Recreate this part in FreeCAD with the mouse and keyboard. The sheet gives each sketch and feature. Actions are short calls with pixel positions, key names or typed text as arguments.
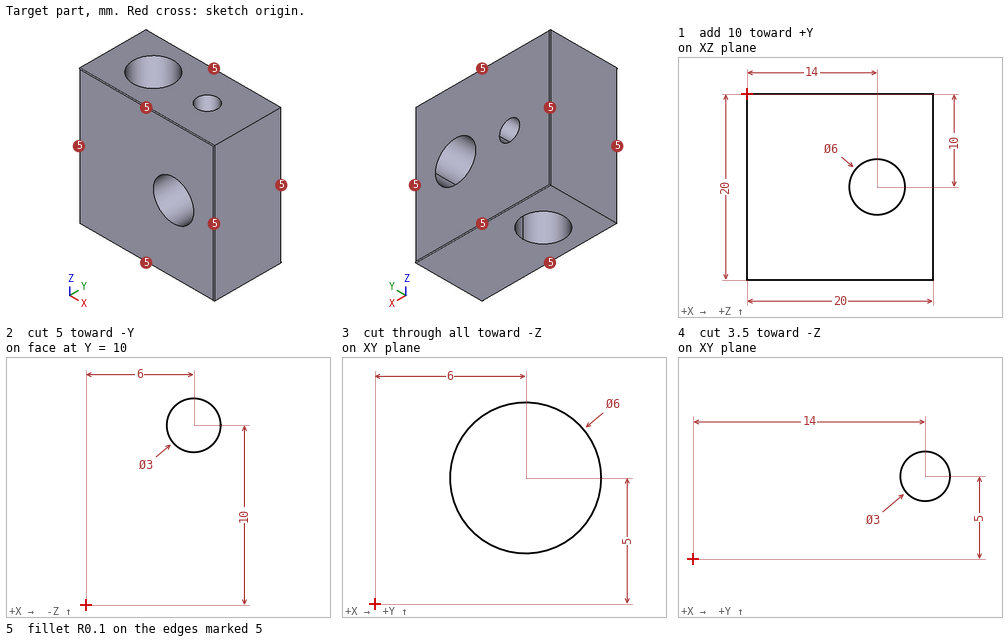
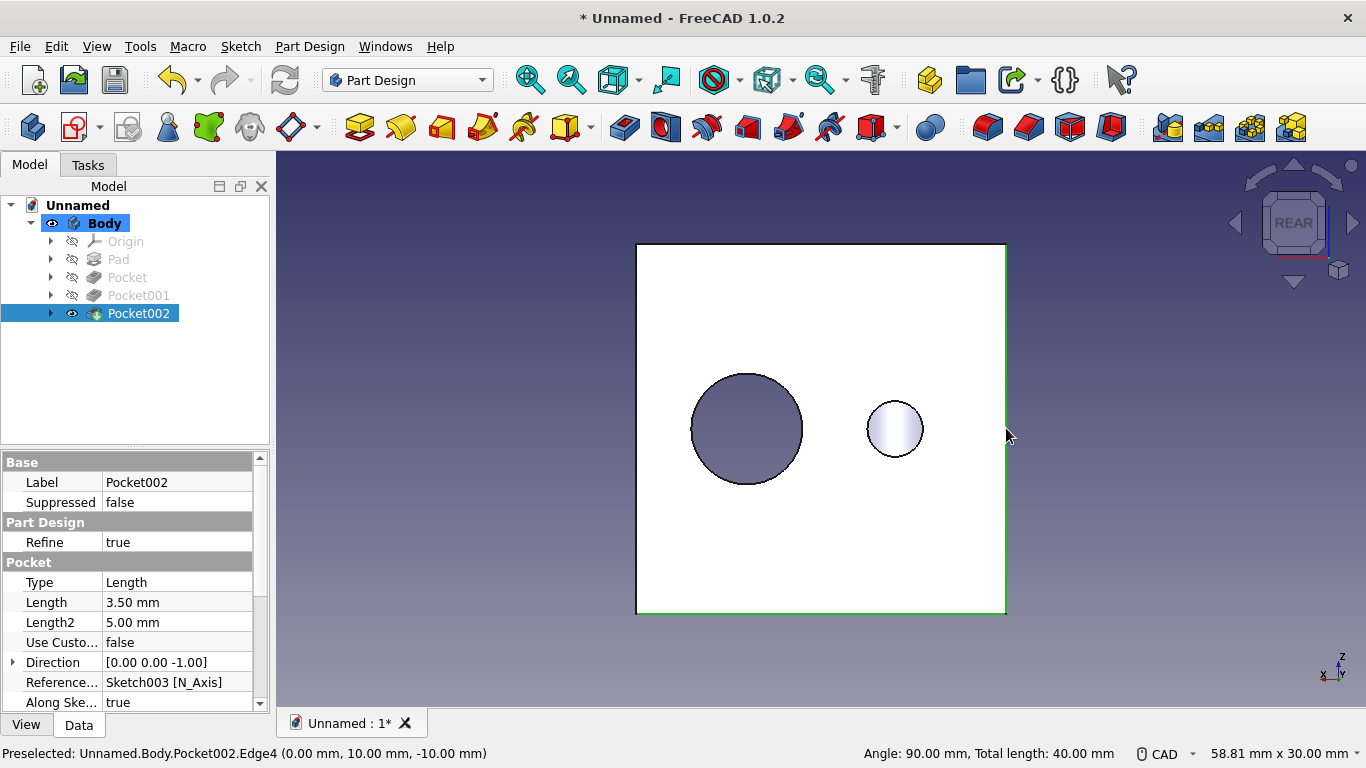
key(0)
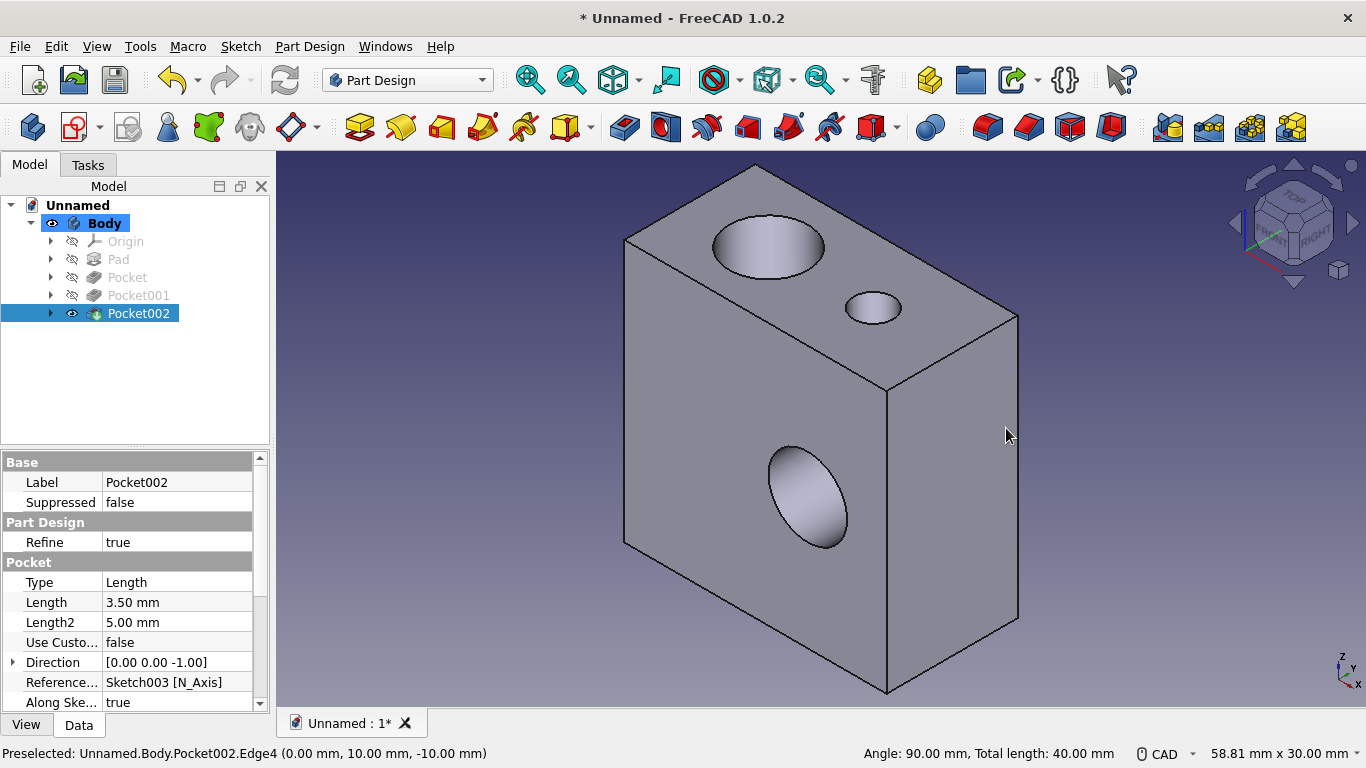
click(887, 541, ctrl)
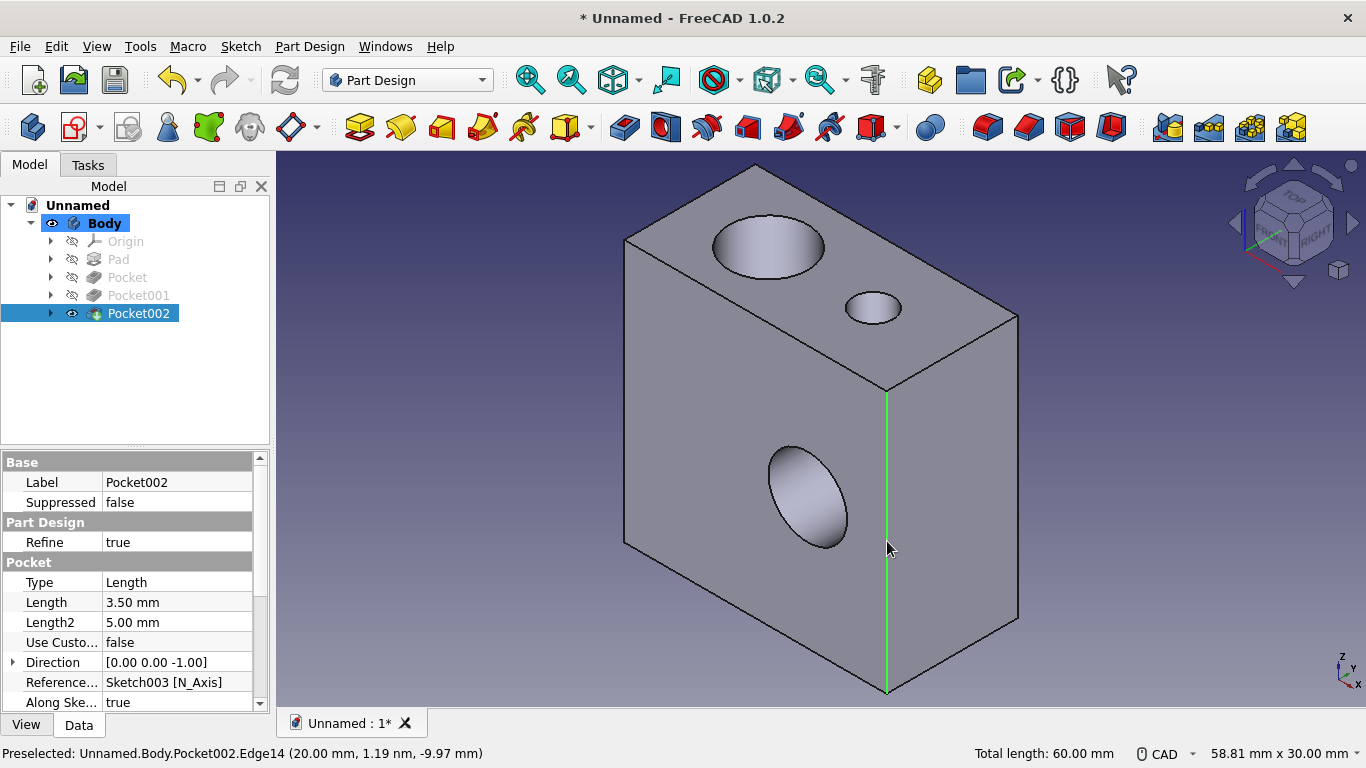
click(755, 315, ctrl)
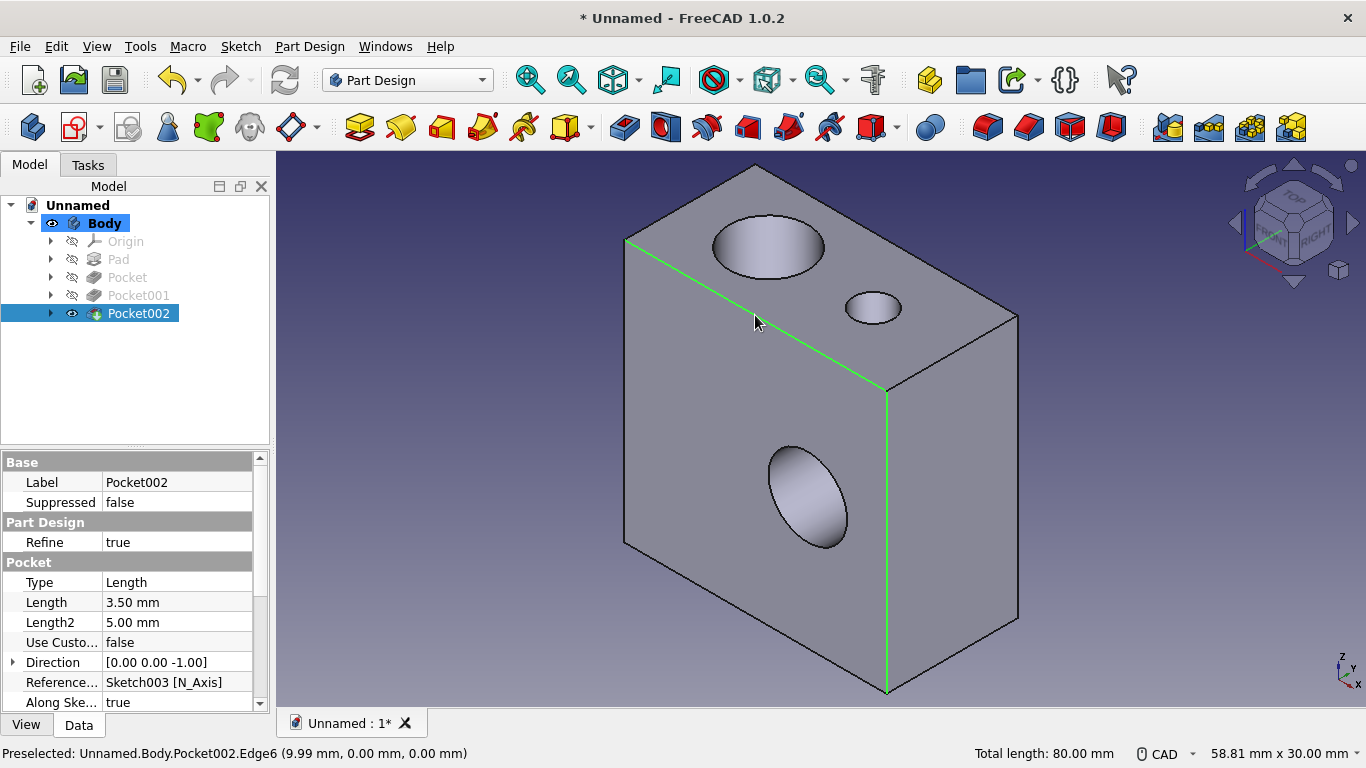
key(2)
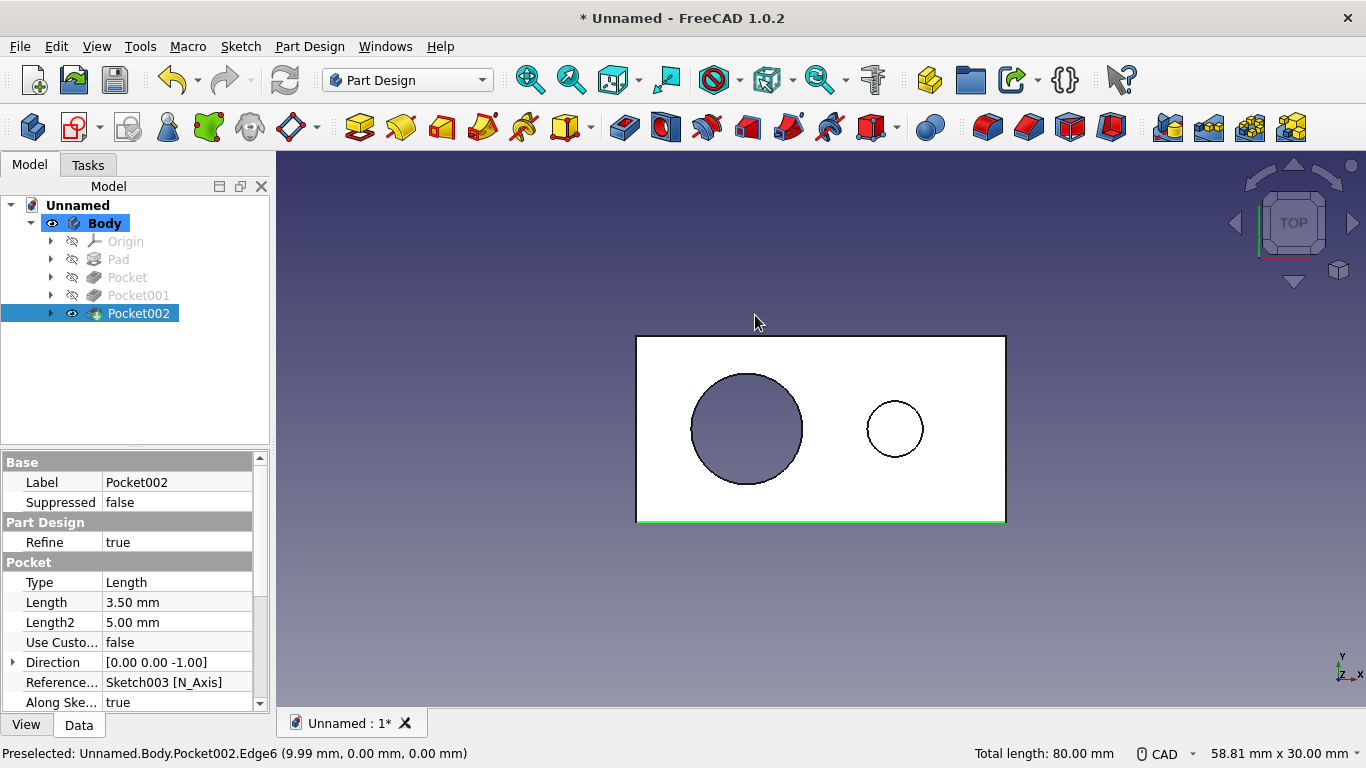
click(531, 80)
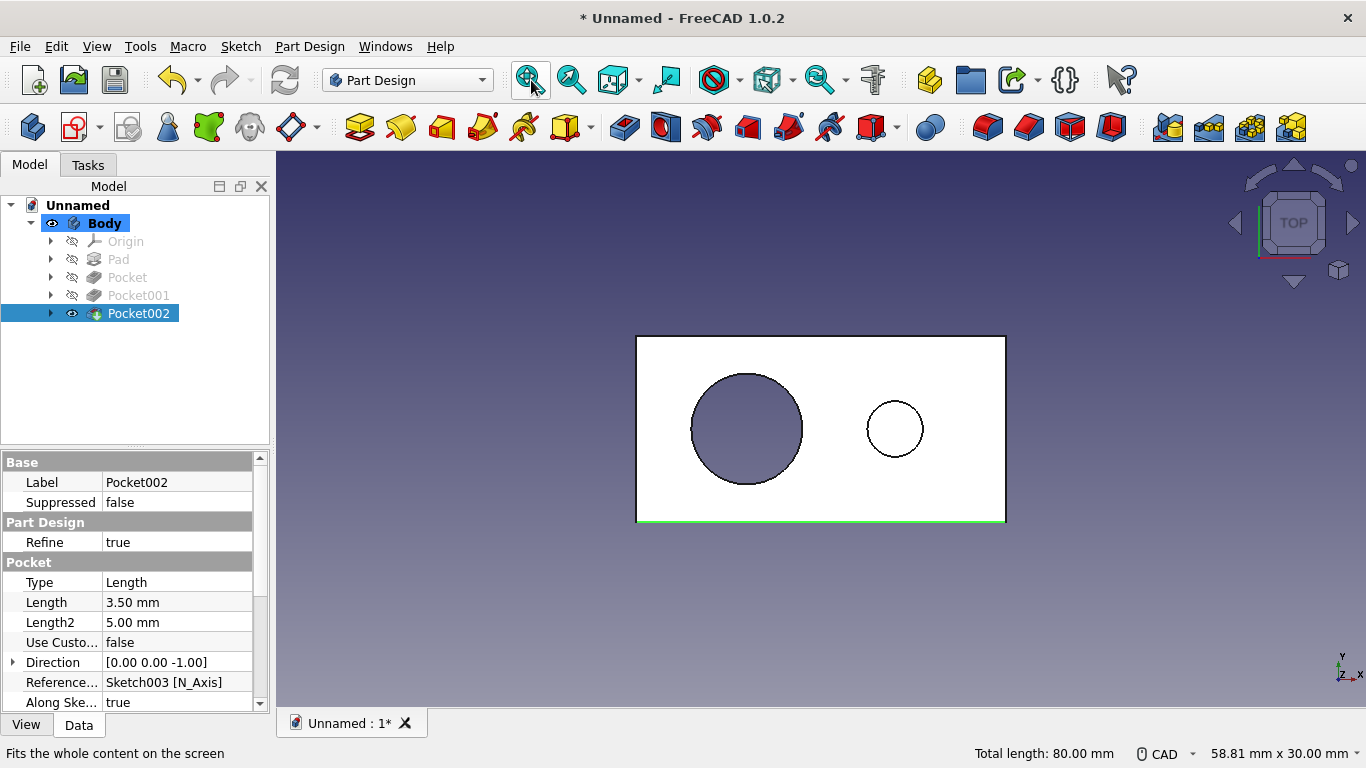
click(821, 335, ctrl)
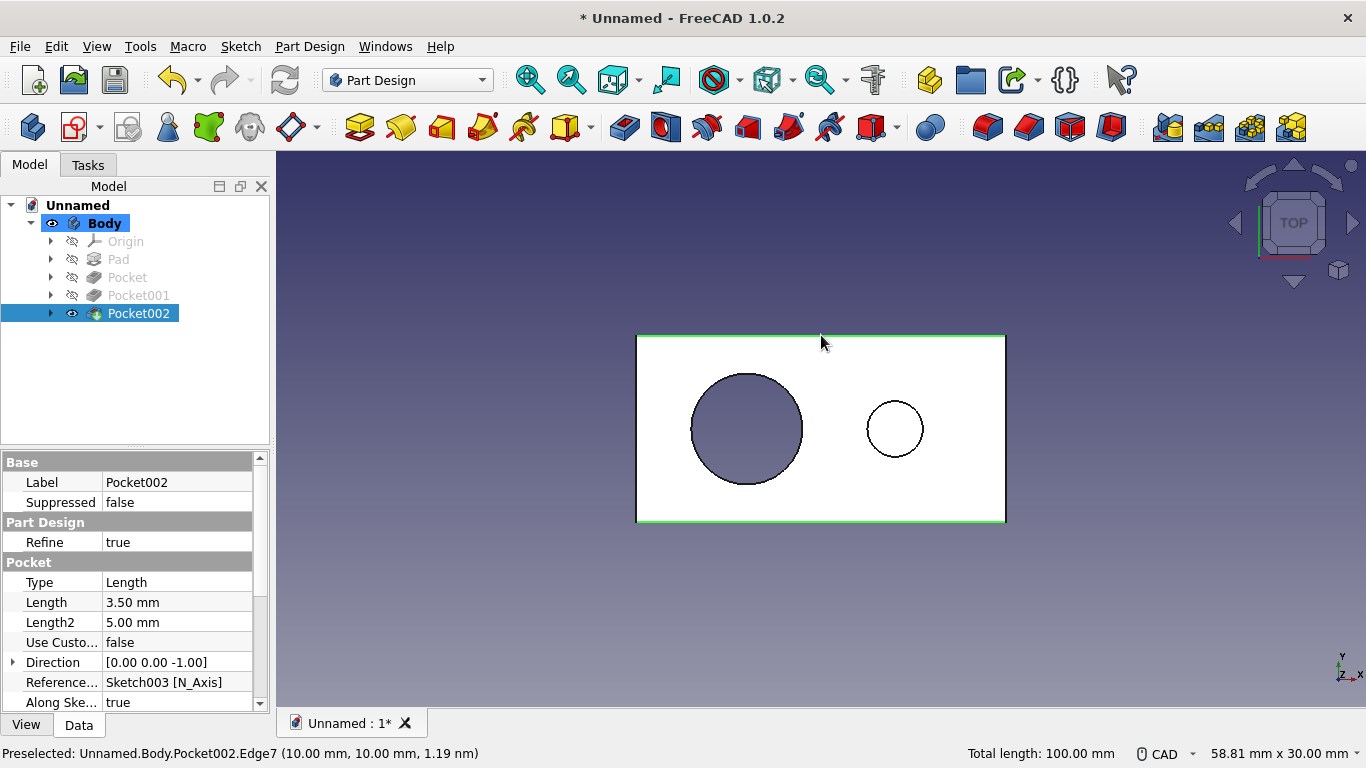
key(1)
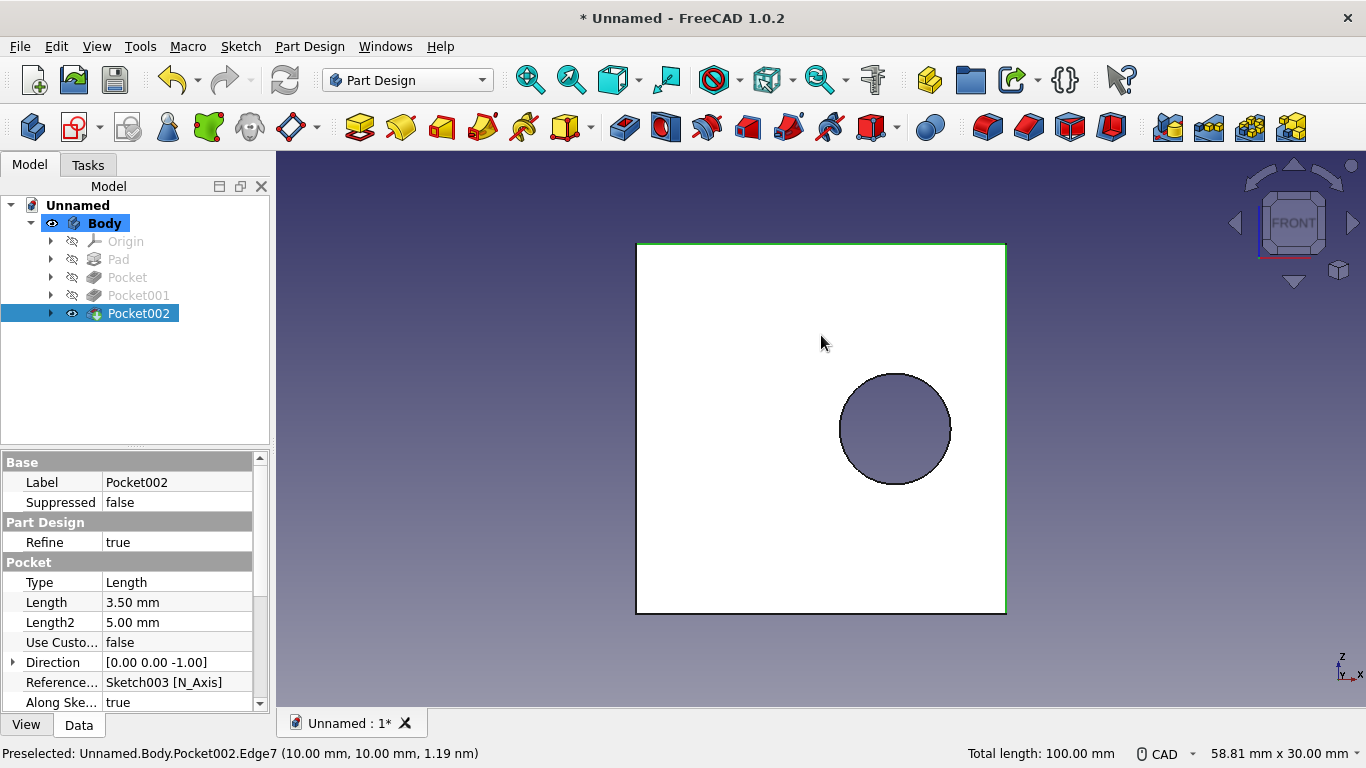
click(636, 391, ctrl)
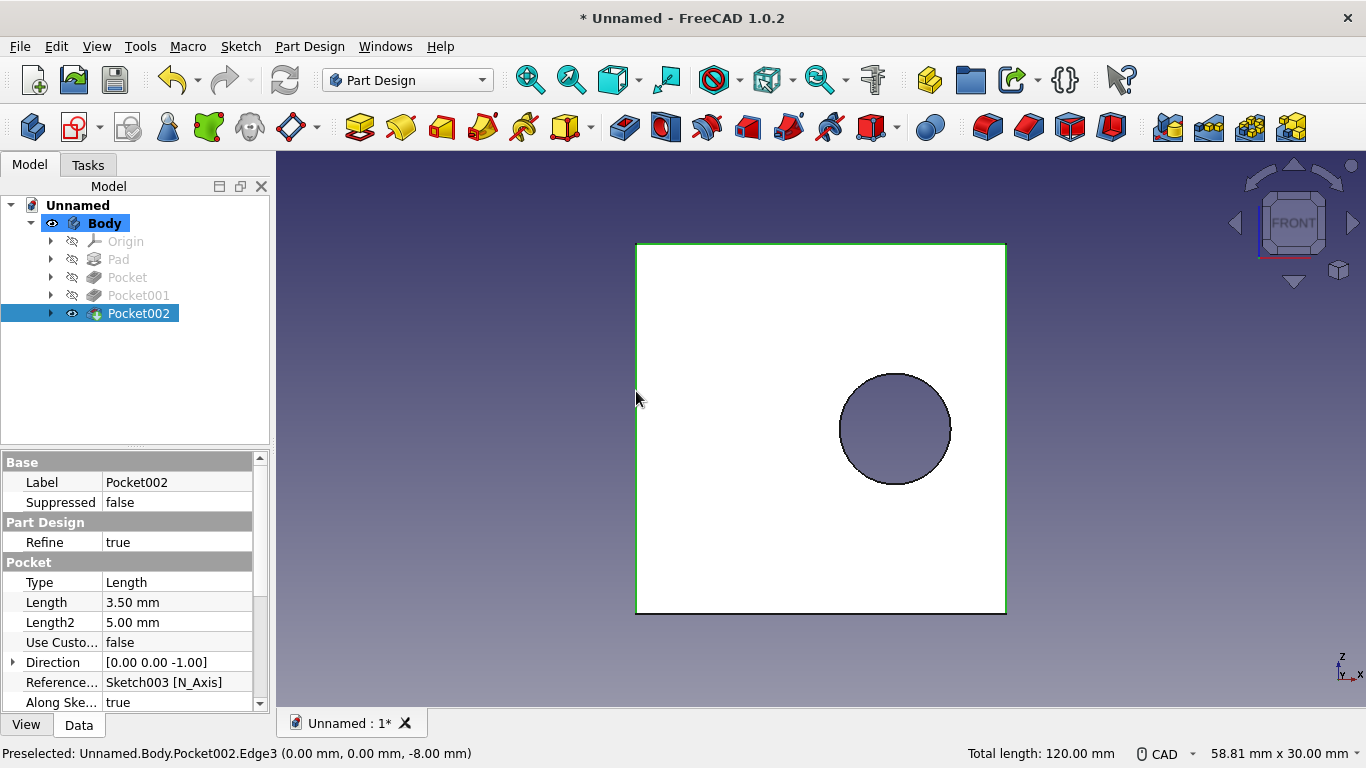
key(3)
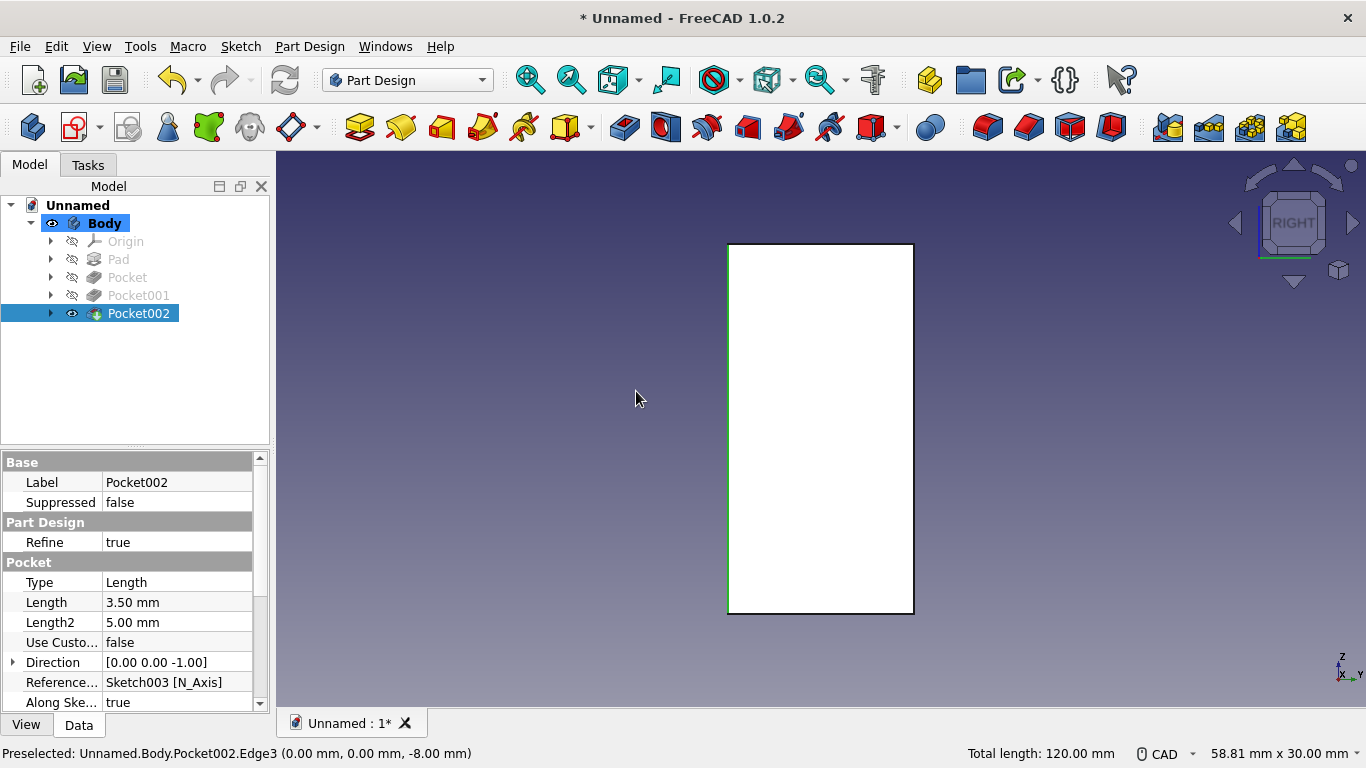
click(914, 428, ctrl)